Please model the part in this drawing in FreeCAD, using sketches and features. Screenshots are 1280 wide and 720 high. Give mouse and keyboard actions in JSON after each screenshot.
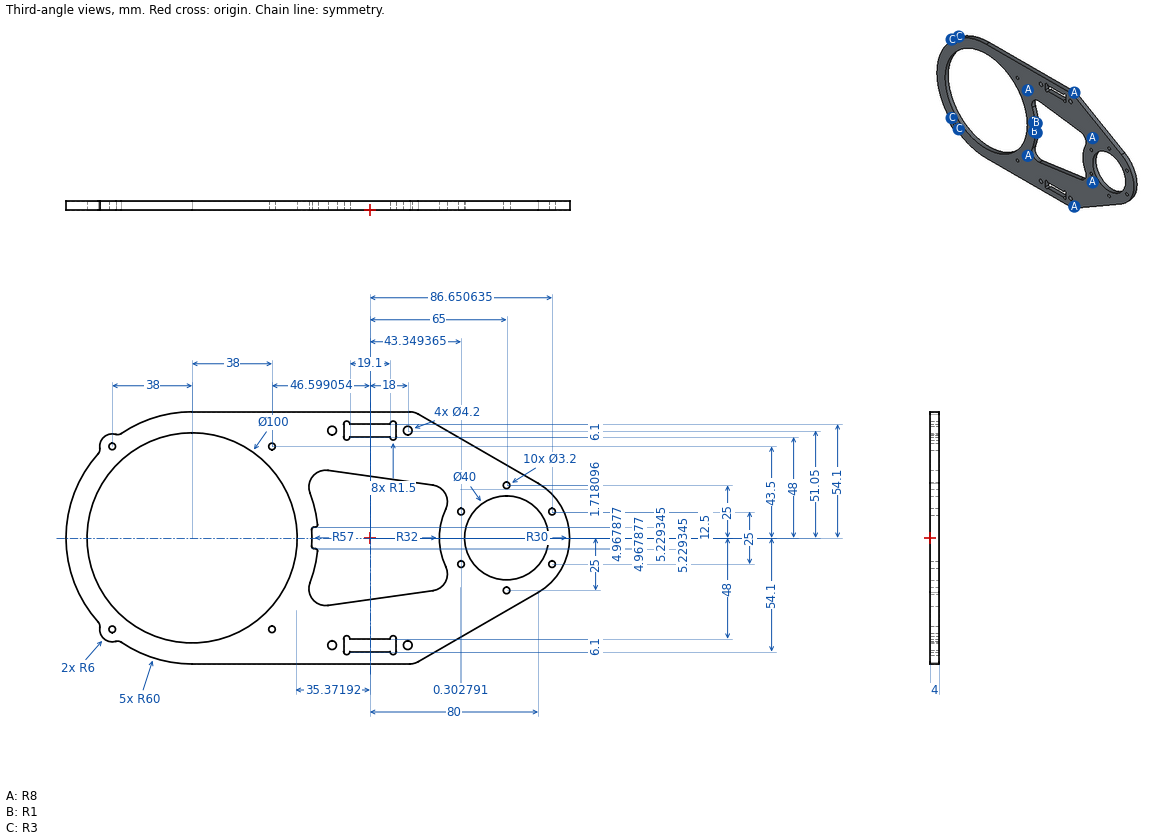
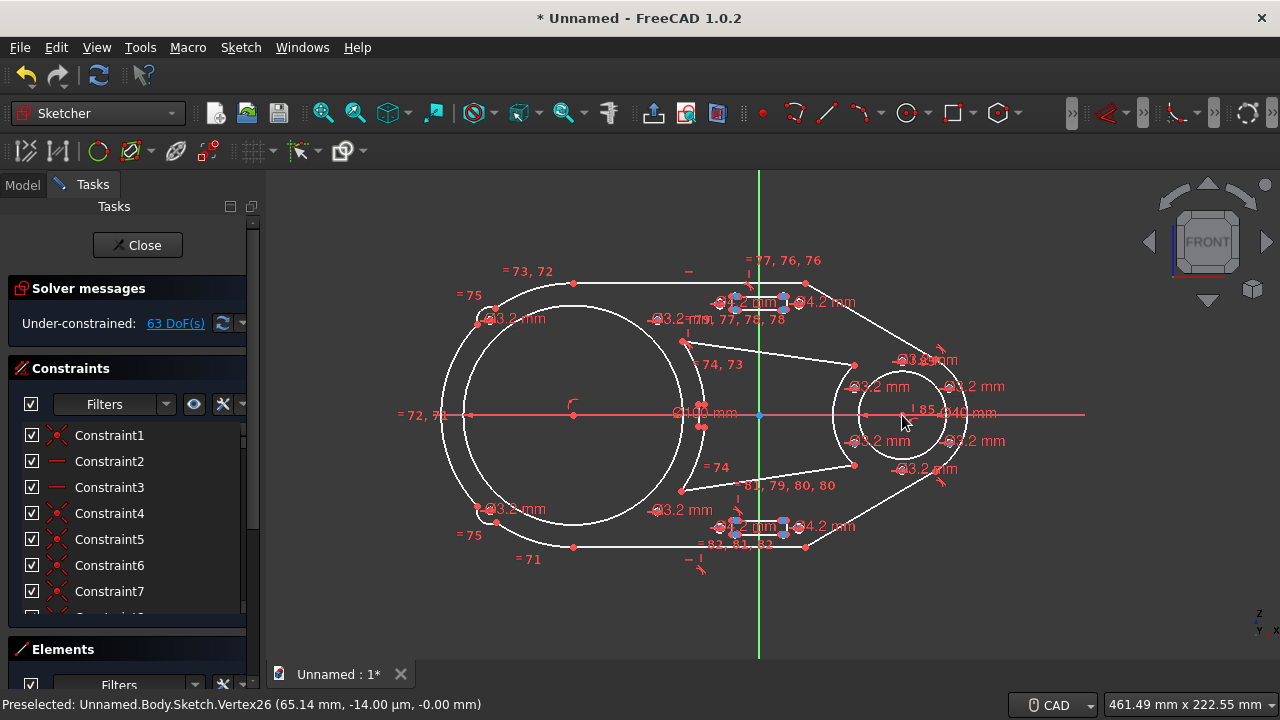
{"action": "left_click", "coordinate": [949, 389]}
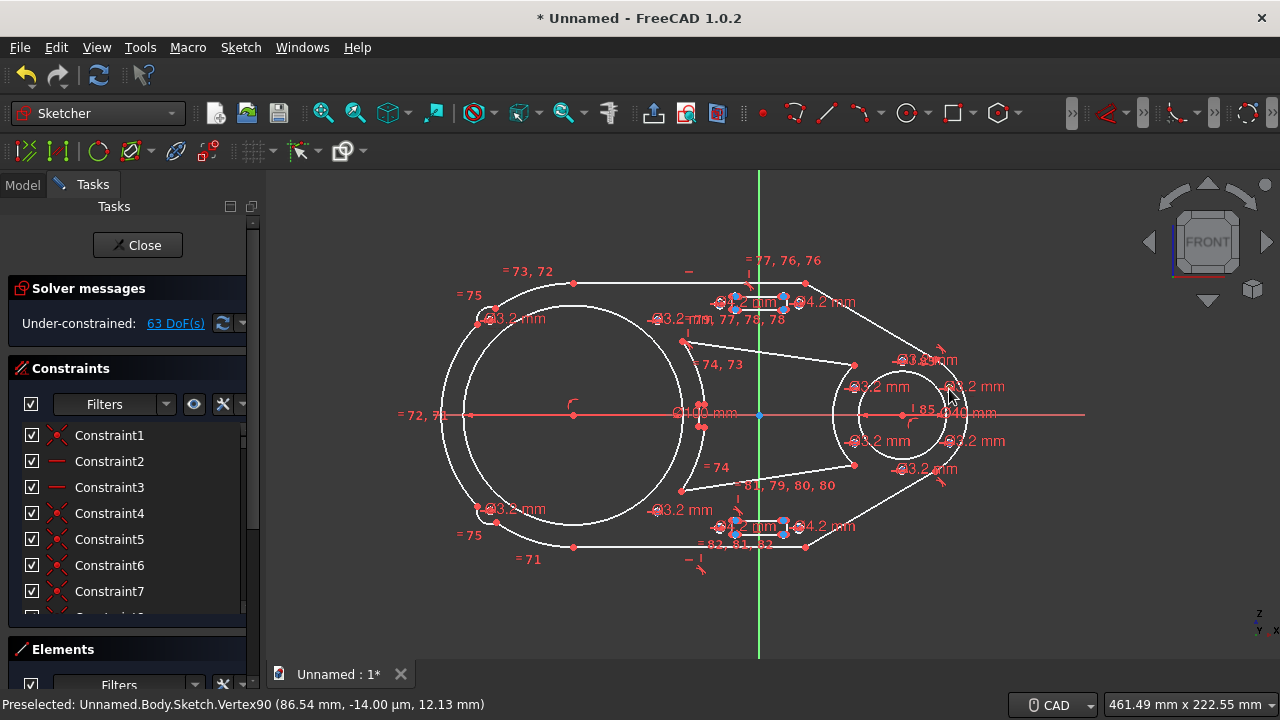
{"action": "left_click", "coordinate": [950, 443]}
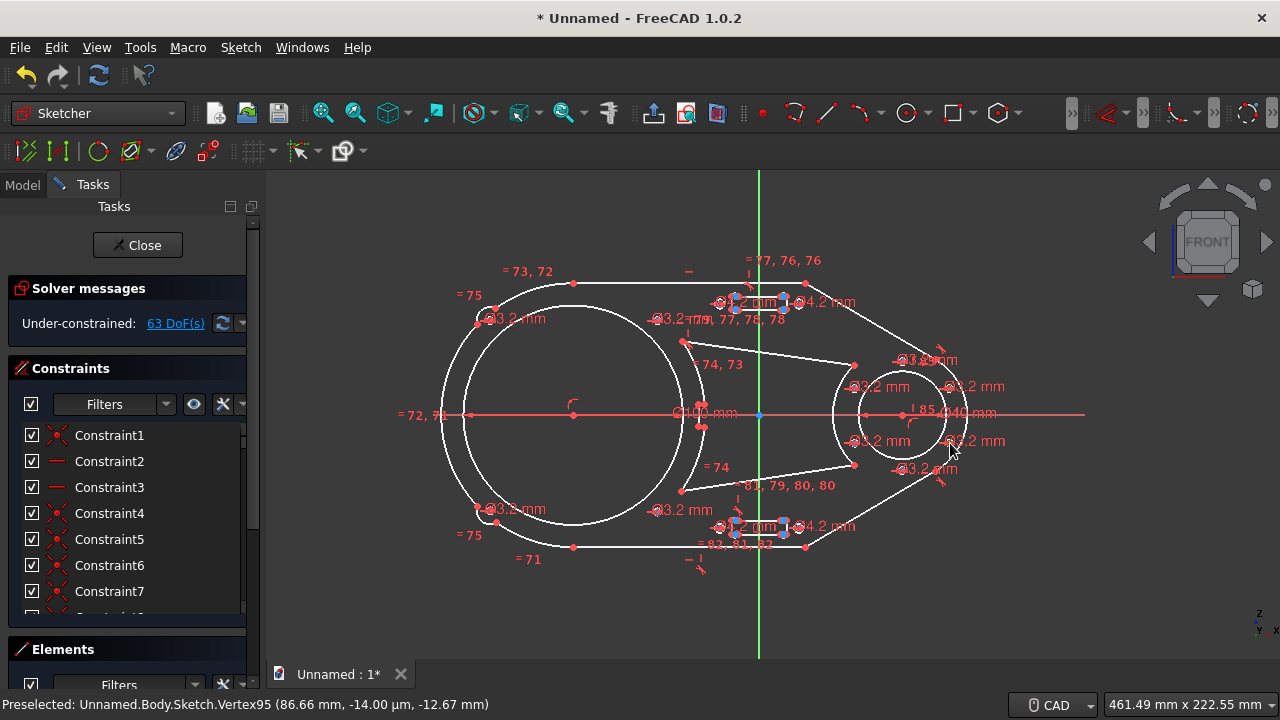
{"action": "key", "text": "v"}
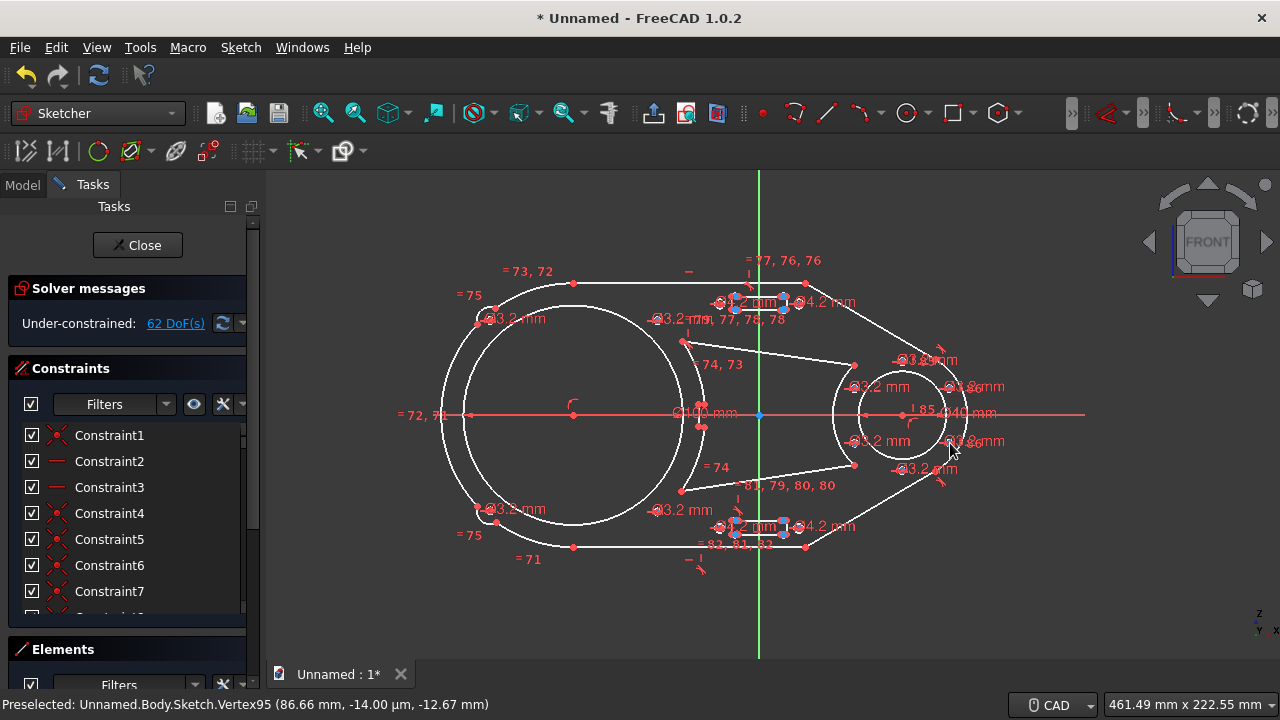
{"action": "left_click", "coordinate": [854, 389]}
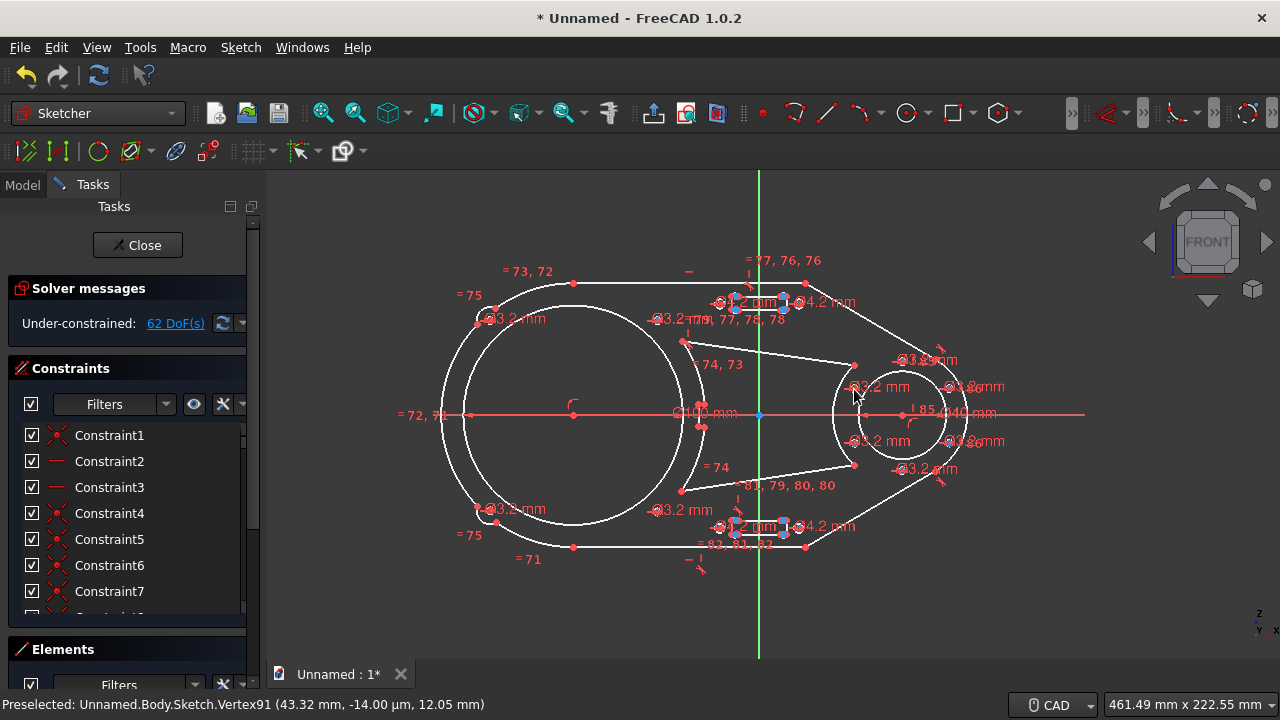
{"action": "left_click", "coordinate": [855, 443]}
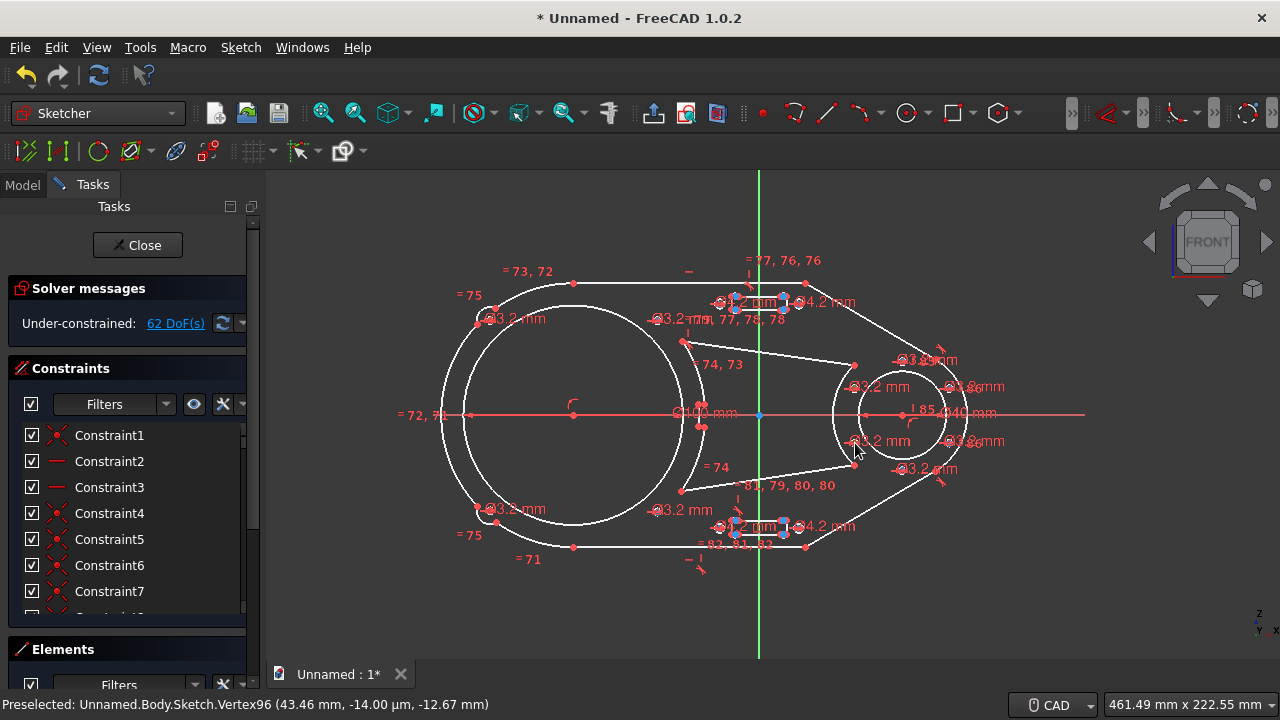
{"action": "key", "text": "v"}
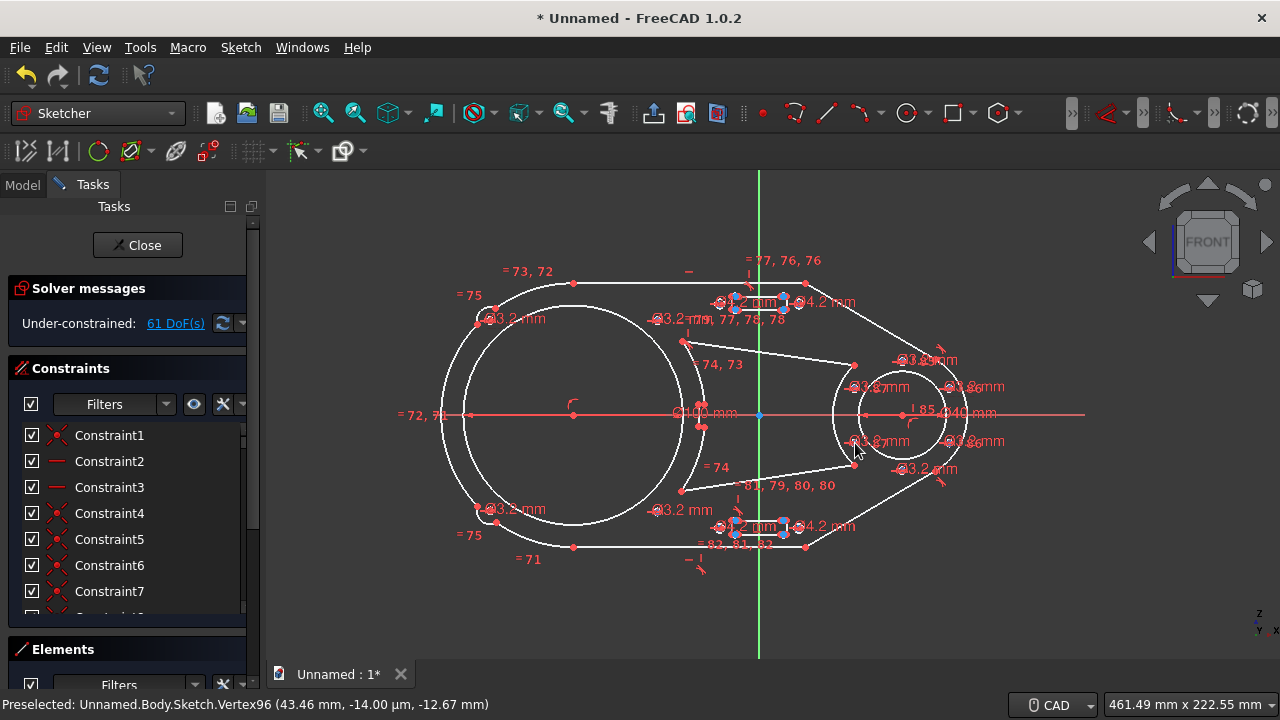
{"action": "left_click", "coordinate": [902, 415]}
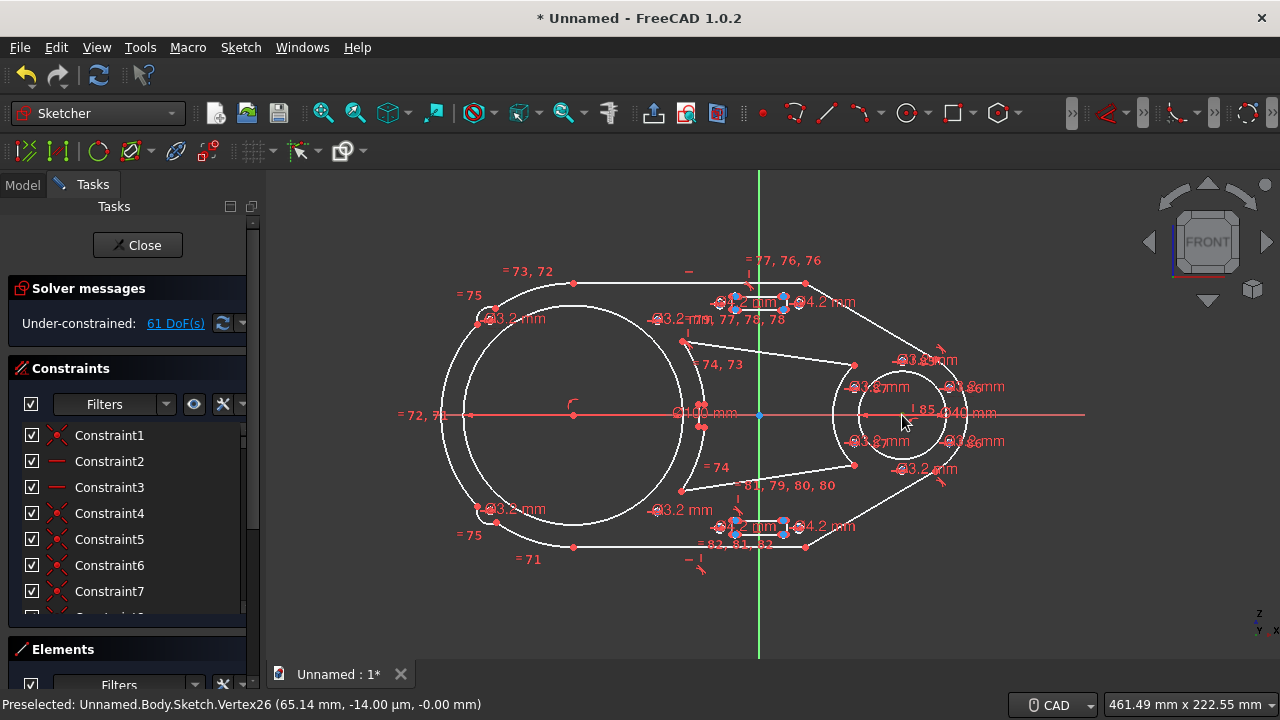
{"action": "left_click", "coordinate": [902, 471]}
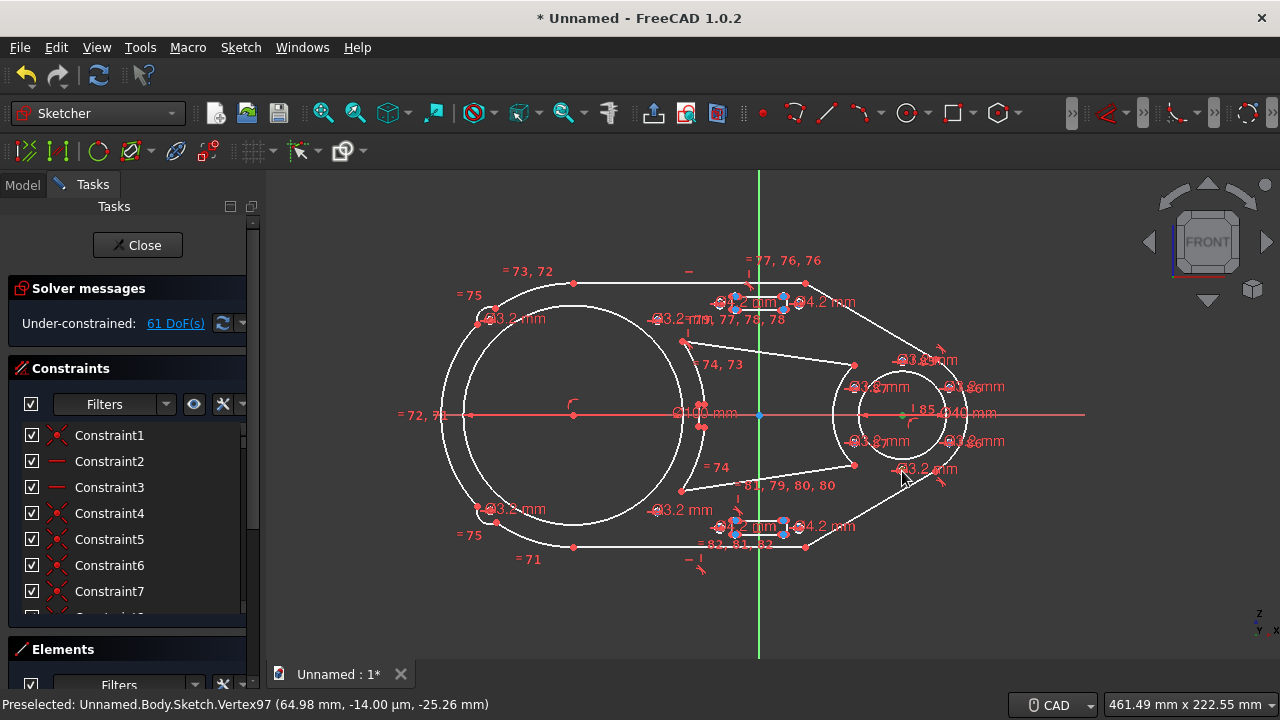
{"action": "key", "text": "v"}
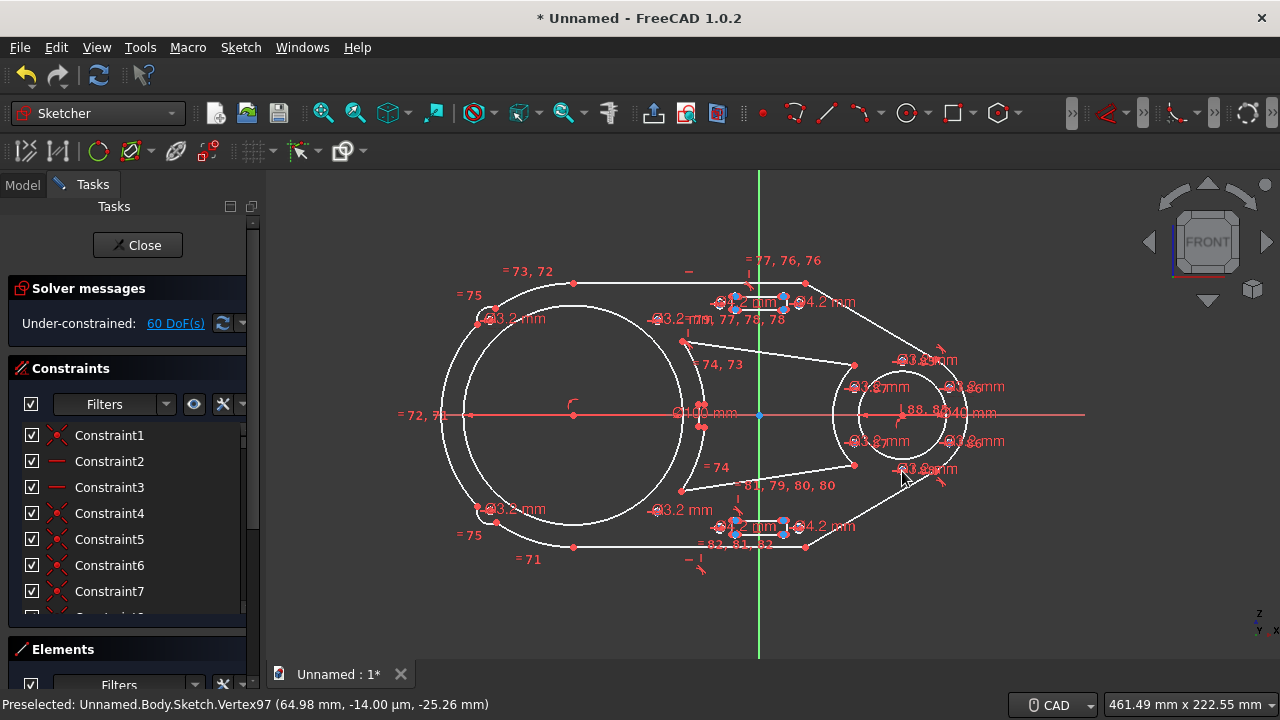
{"action": "left_click", "coordinate": [490, 511]}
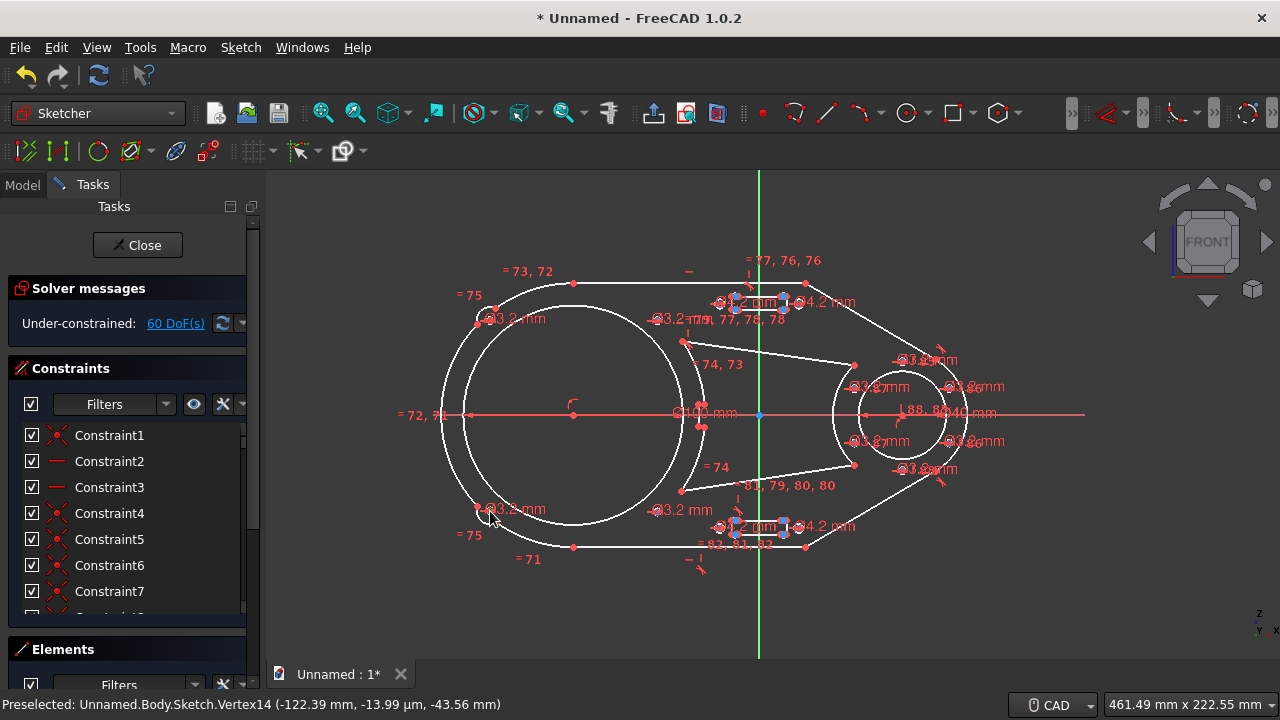
{"action": "left_click", "coordinate": [490, 321]}